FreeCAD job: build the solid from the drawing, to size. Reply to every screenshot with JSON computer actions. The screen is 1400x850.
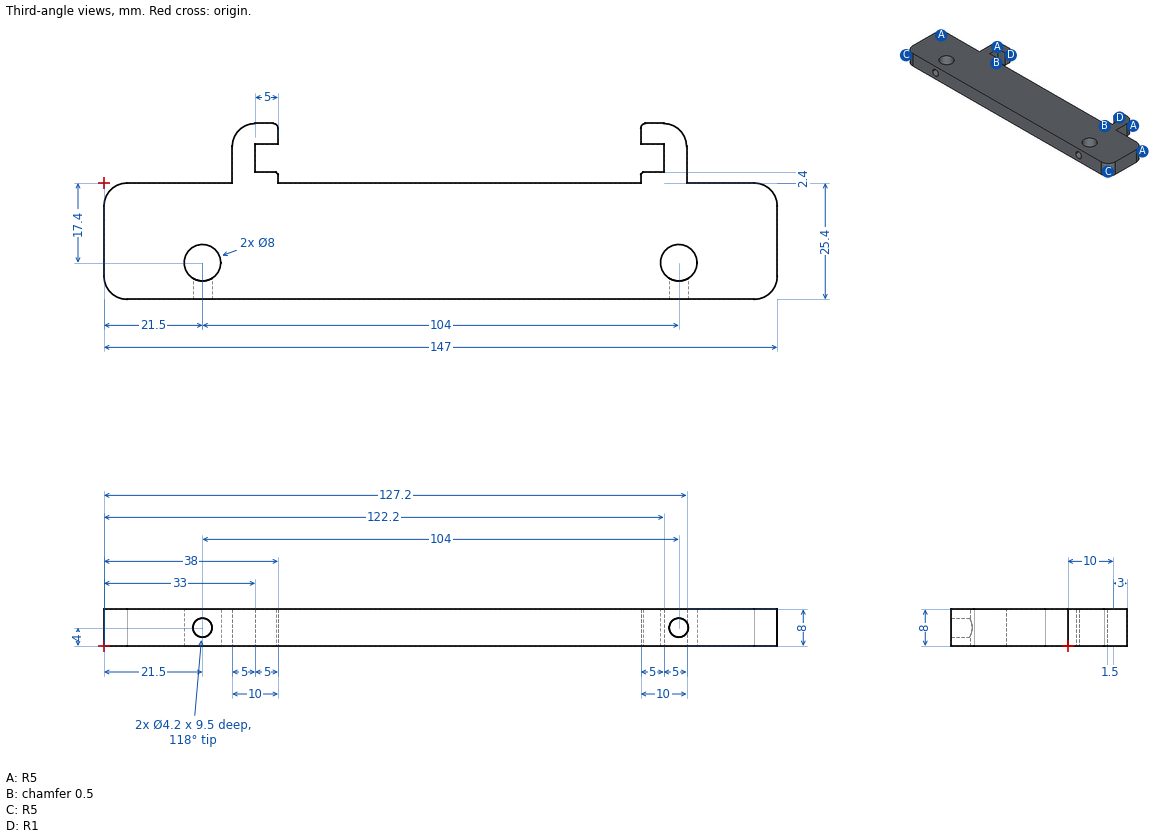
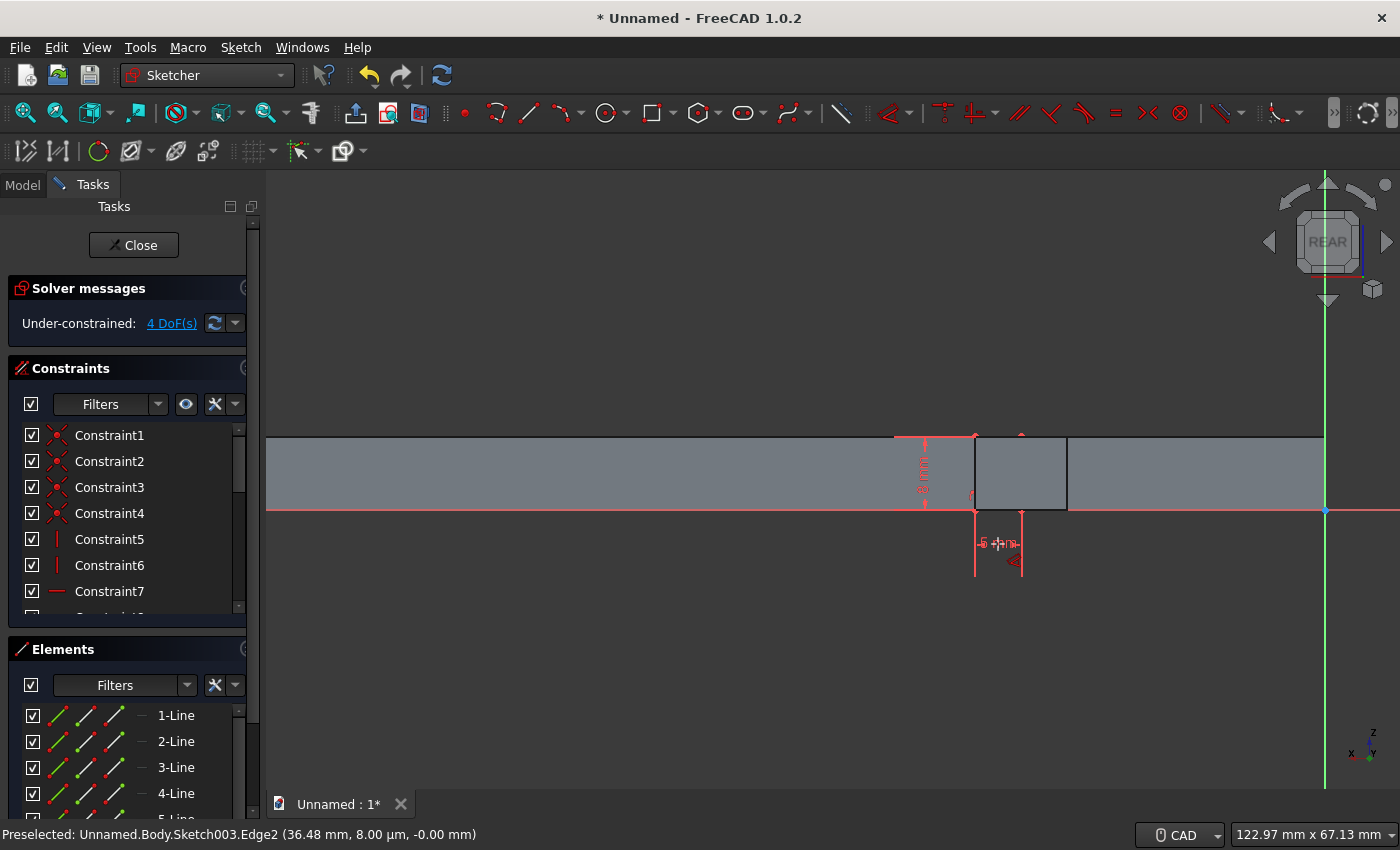
{"action": "scroll", "coordinate": [768, 487], "scroll_direction": "down", "scroll_amount": 3}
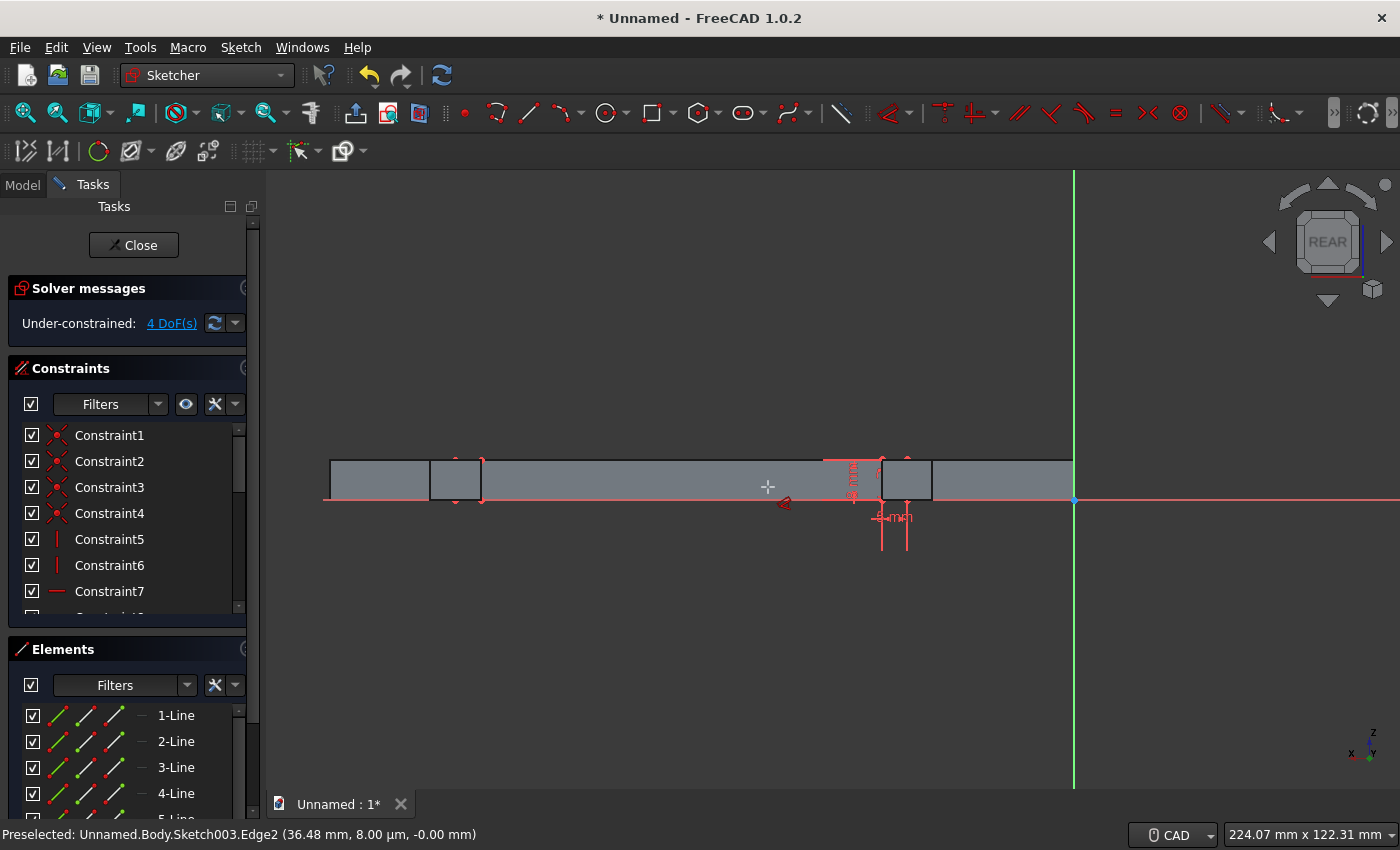
{"action": "left_click", "coordinate": [455, 473]}
{"action": "left_click", "coordinate": [421, 480]}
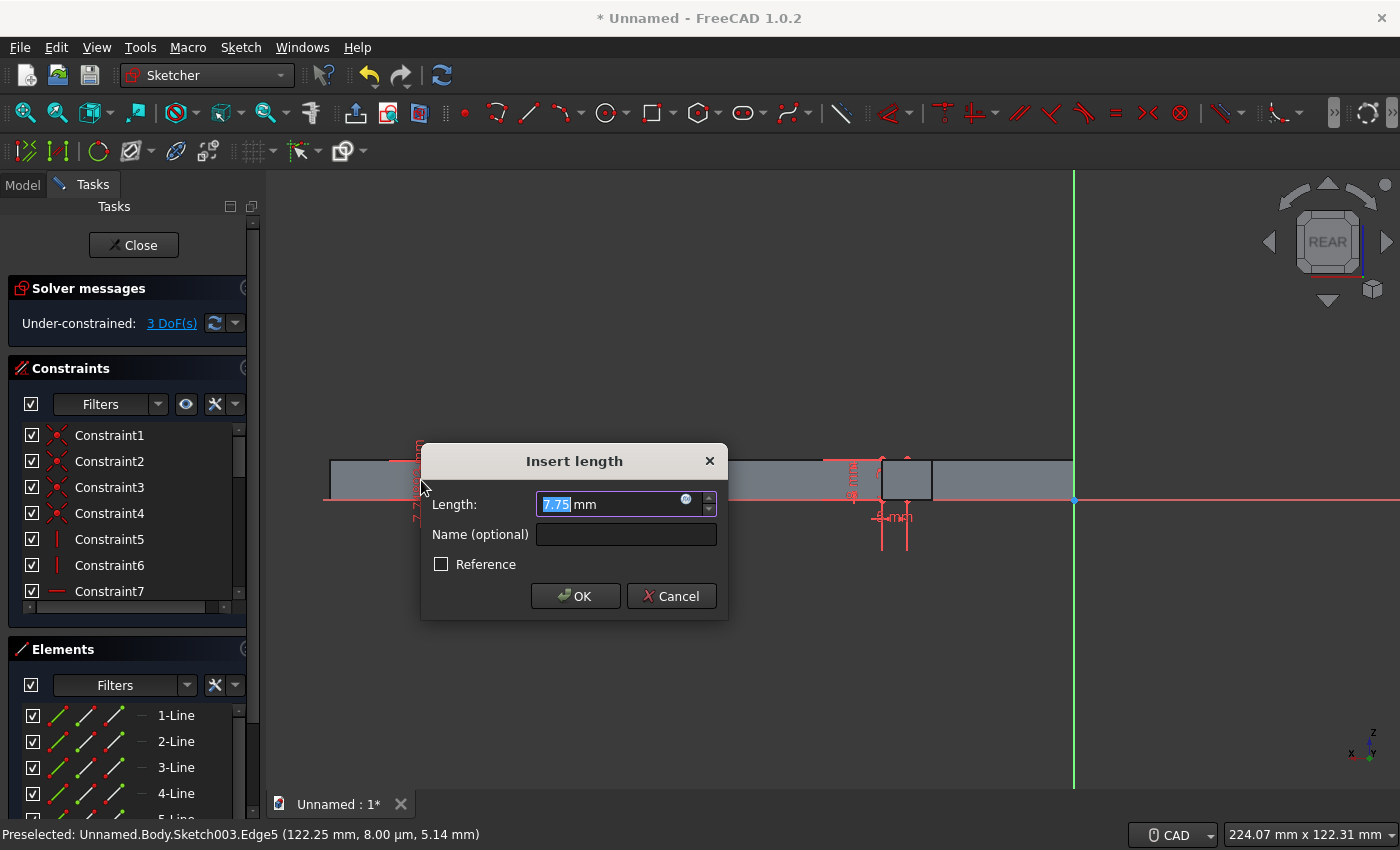
{"action": "type", "text": "8"}
{"action": "key", "text": "Return"}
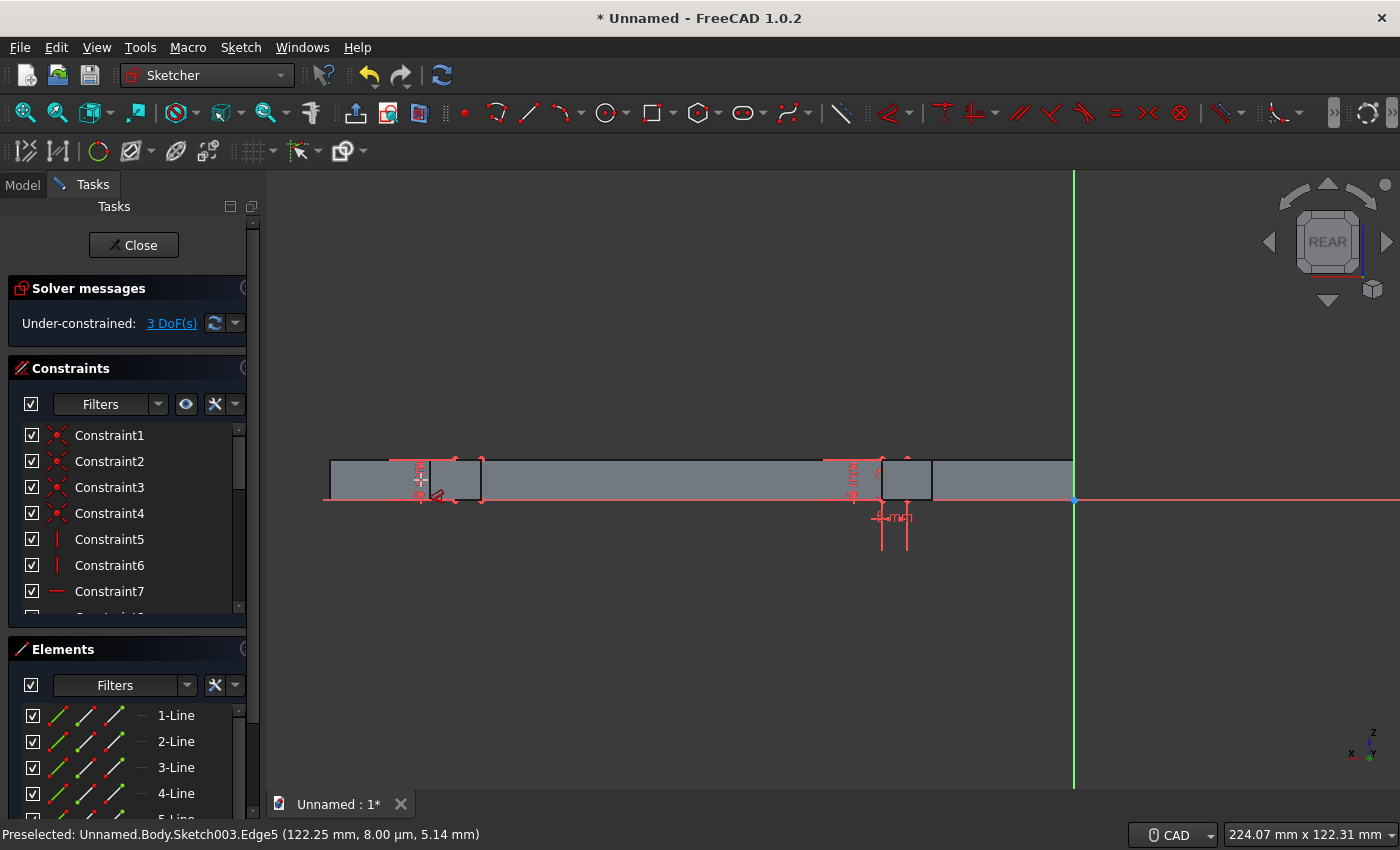
{"action": "scroll", "coordinate": [466, 500], "scroll_direction": "up", "scroll_amount": 3}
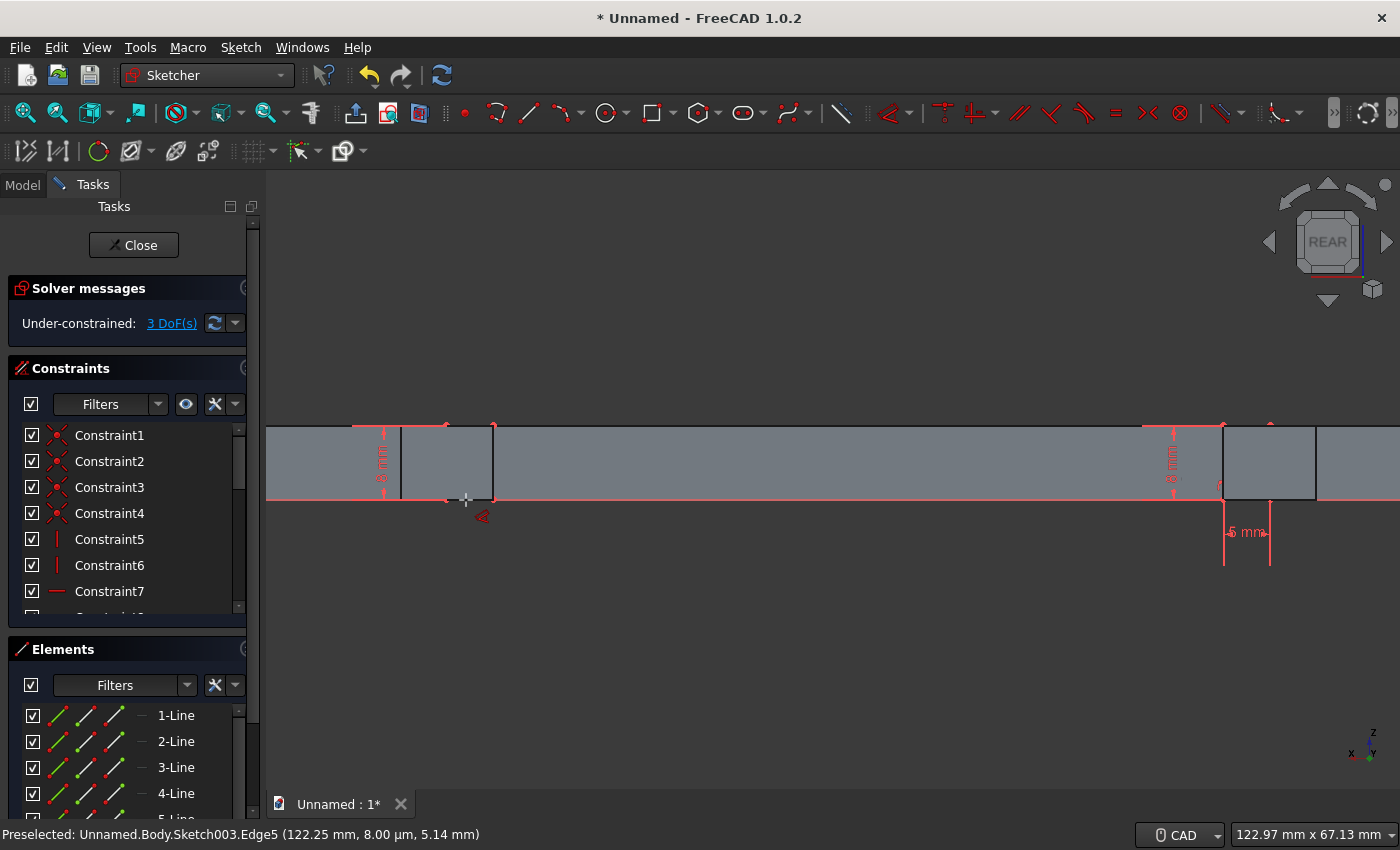
{"action": "left_click", "coordinate": [465, 500]}
{"action": "left_click", "coordinate": [470, 534]}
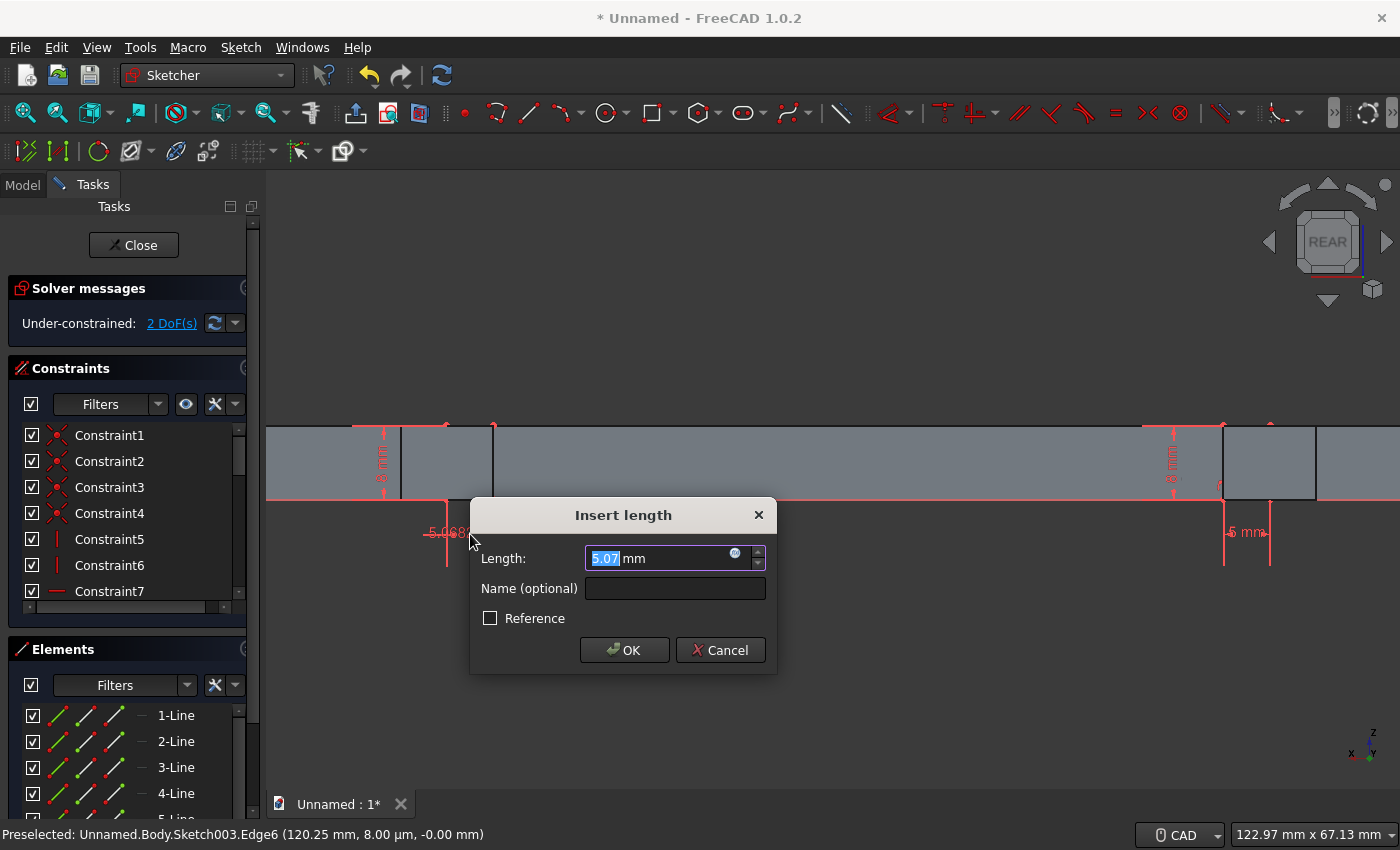
{"action": "type", "text": "5"}
{"action": "key", "text": "Return"}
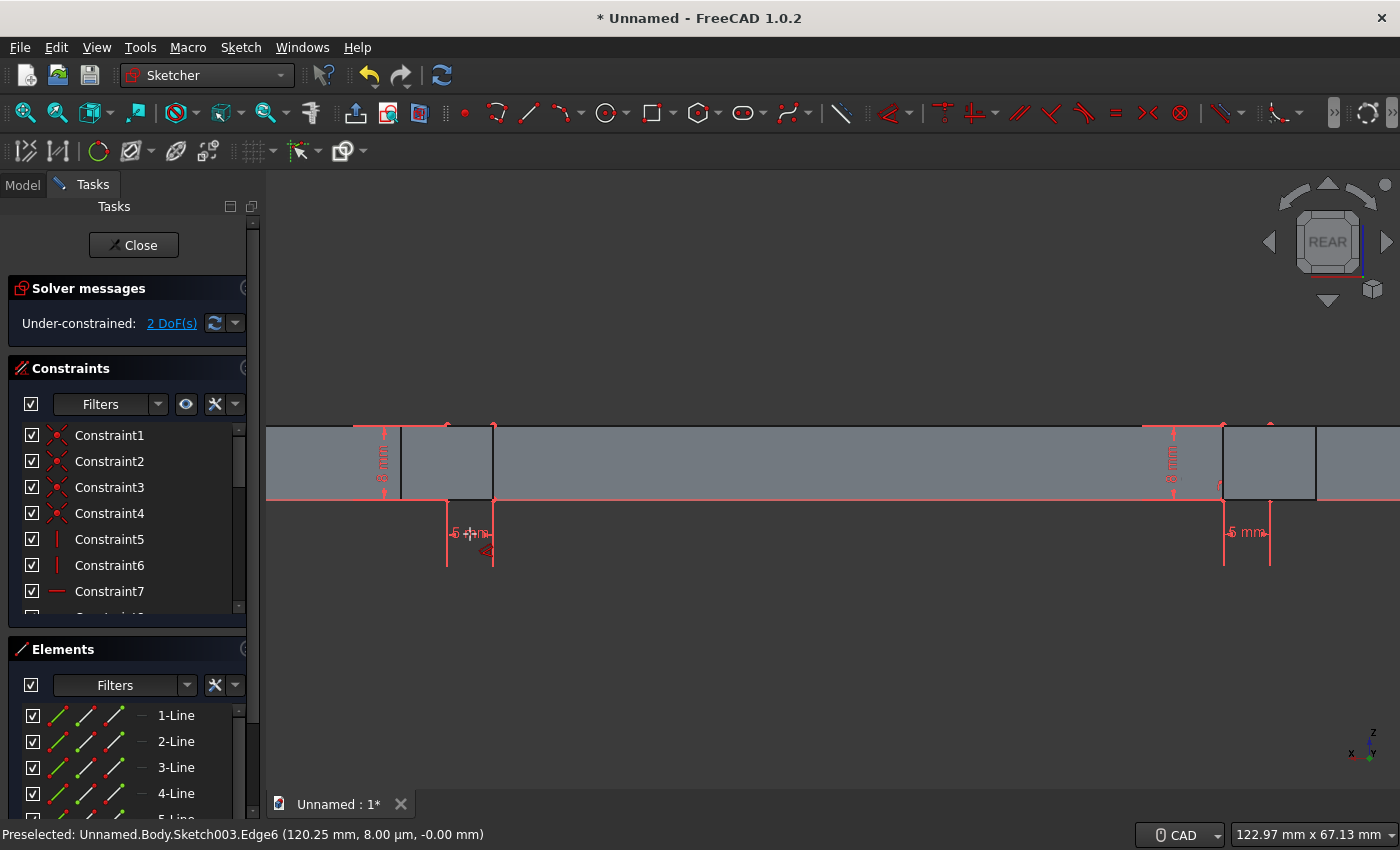
{"action": "left_click", "coordinate": [1224, 426]}
{"action": "left_click", "coordinate": [1229, 392]}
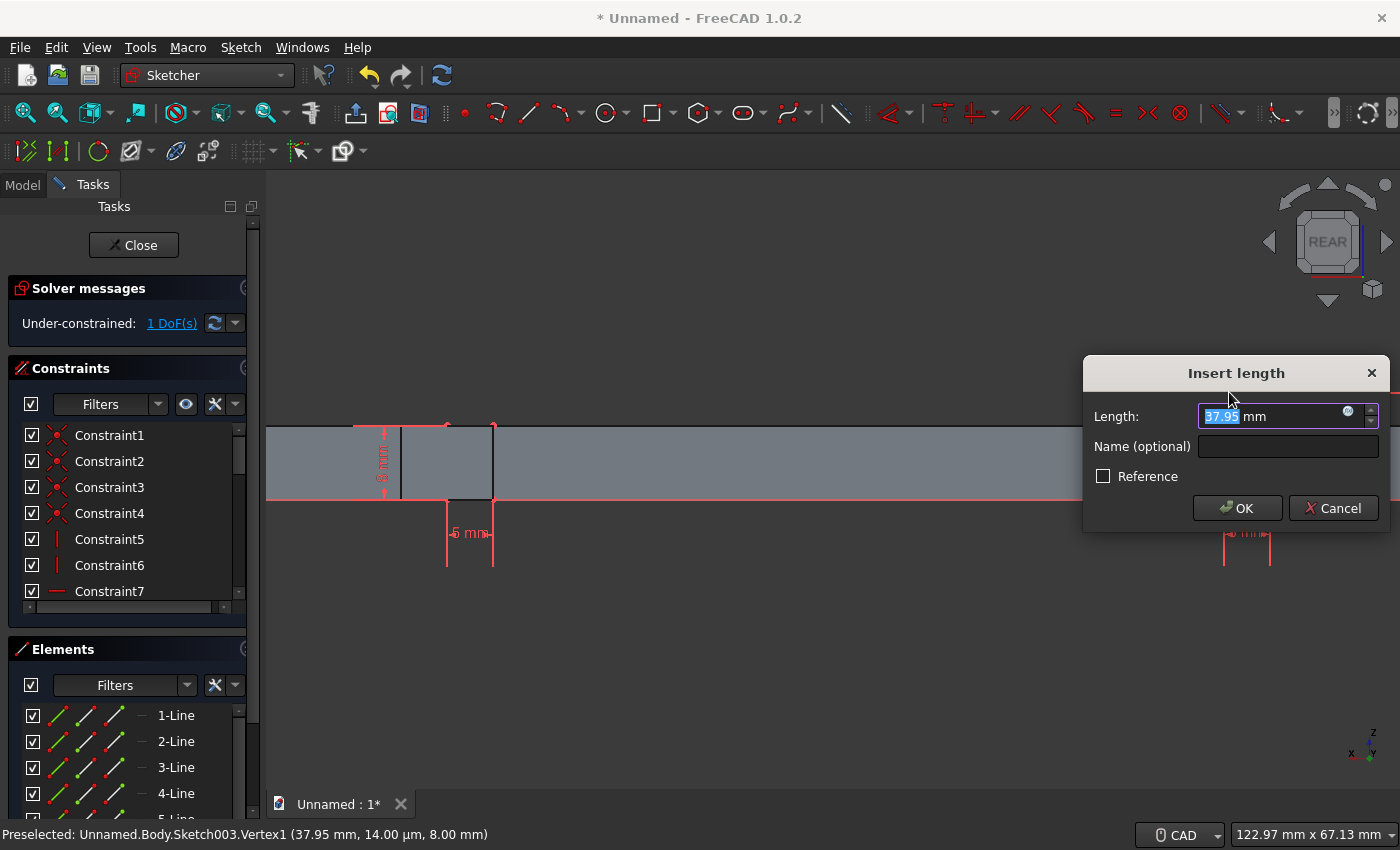
{"action": "type", "text": "38"}
{"action": "key", "text": "Return"}